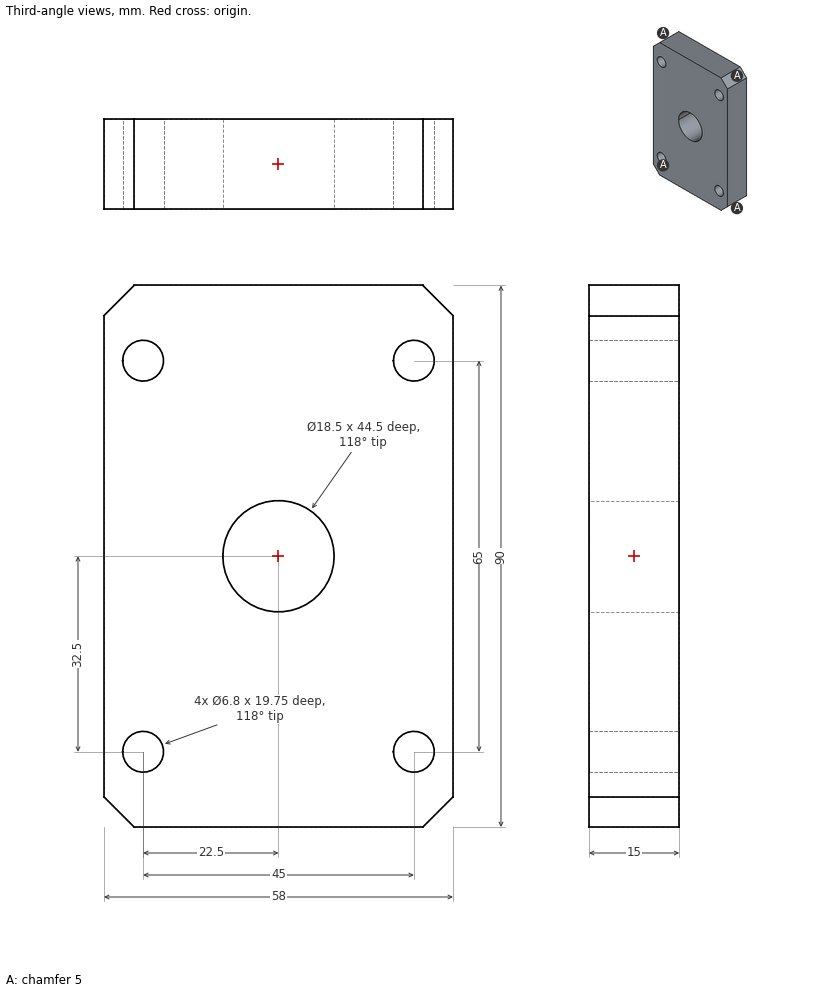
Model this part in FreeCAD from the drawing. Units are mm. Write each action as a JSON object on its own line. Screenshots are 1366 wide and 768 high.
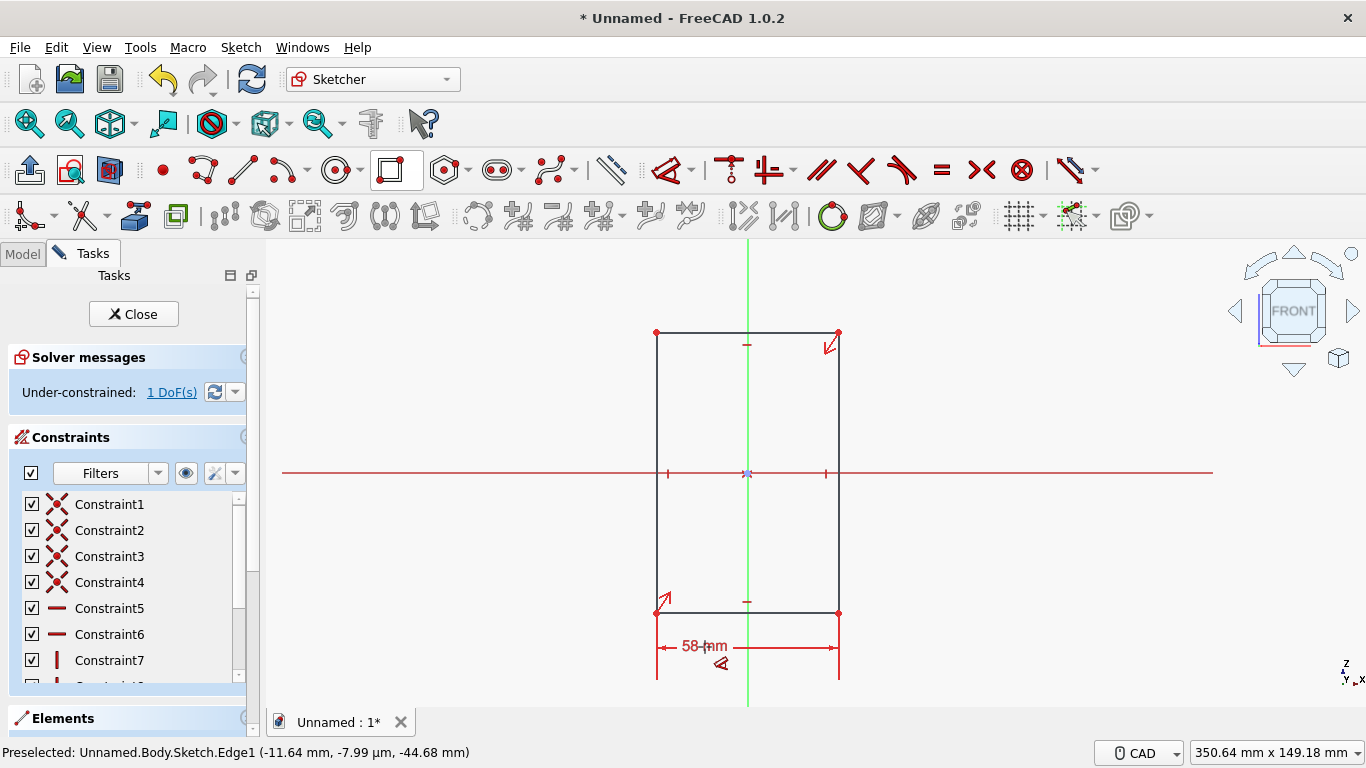
{"action": "left_click", "coordinate": [839, 529]}
{"action": "left_click", "coordinate": [873, 409]}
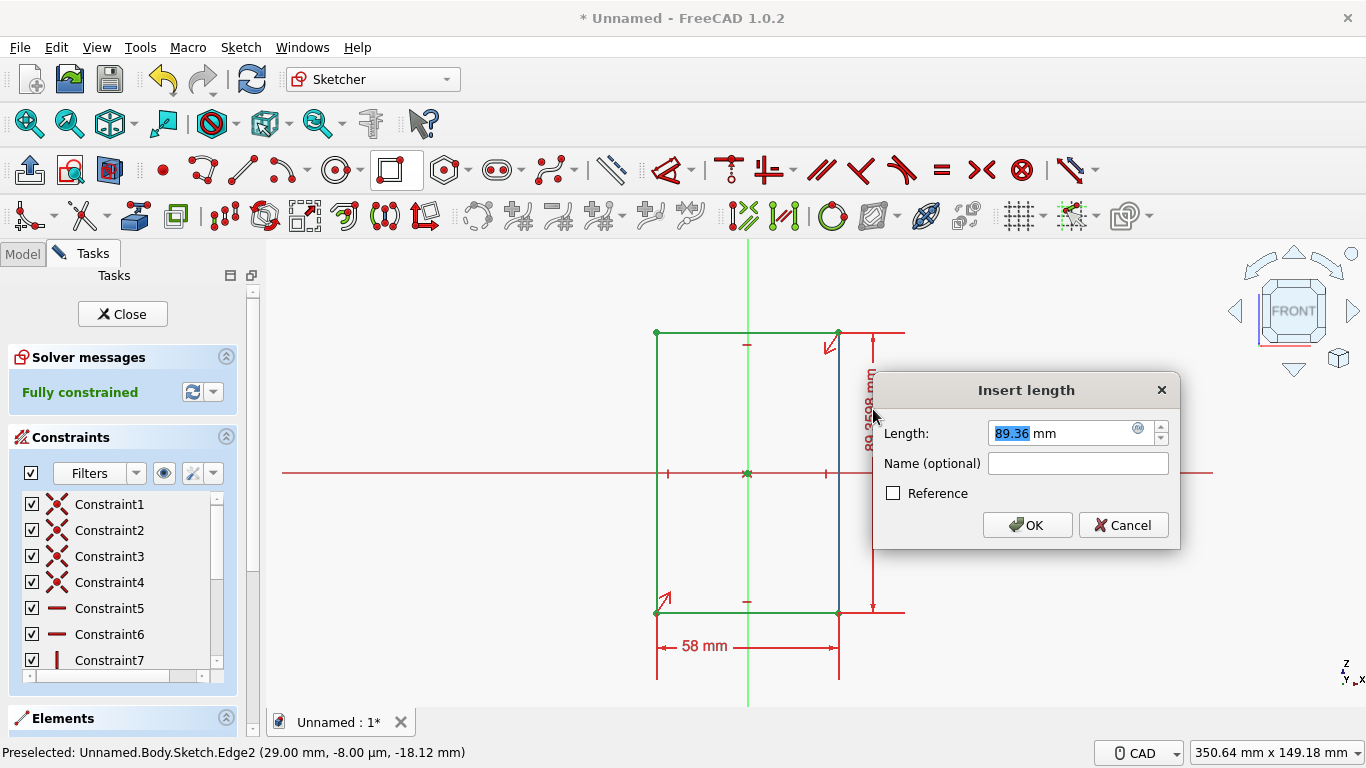
{"action": "type", "text": "90"}
{"action": "key", "text": "Return"}
{"action": "key", "text": "Escape"}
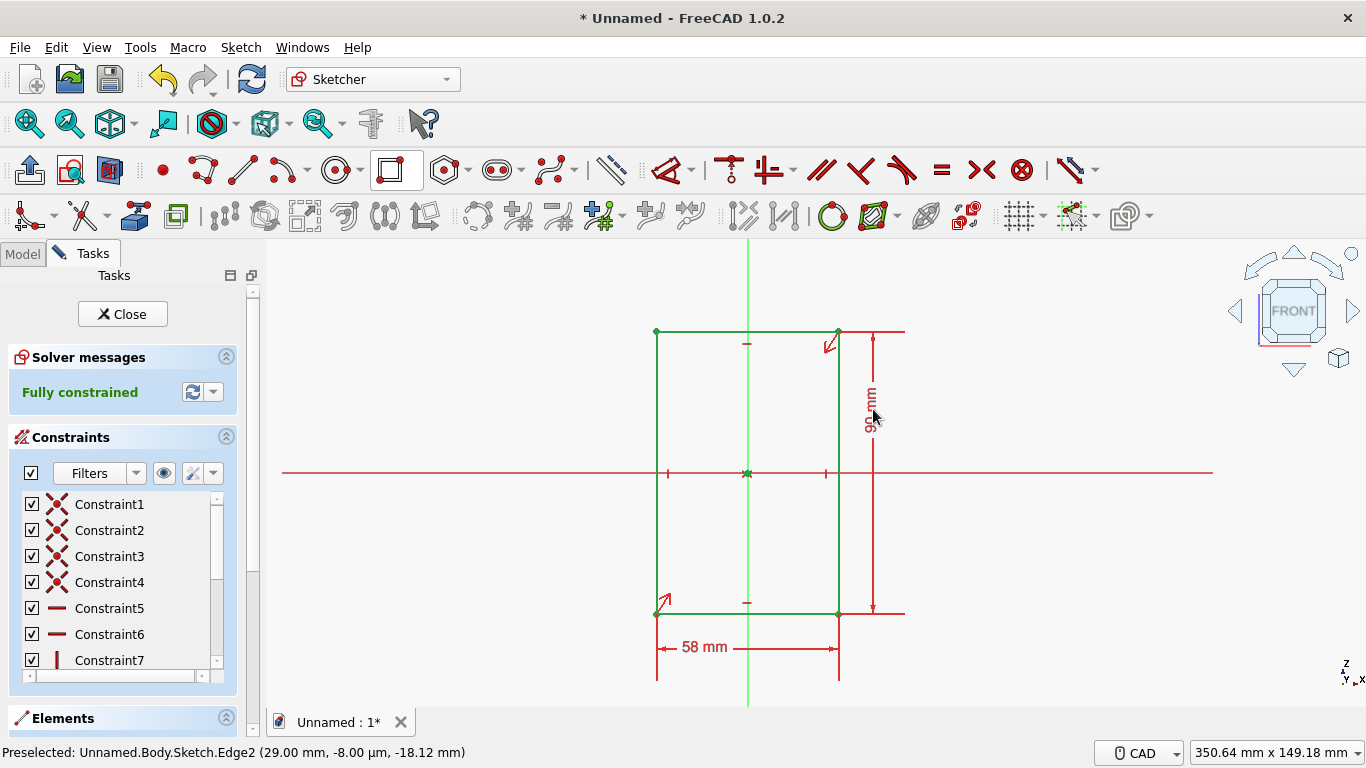
{"action": "left_click", "coordinate": [123, 314]}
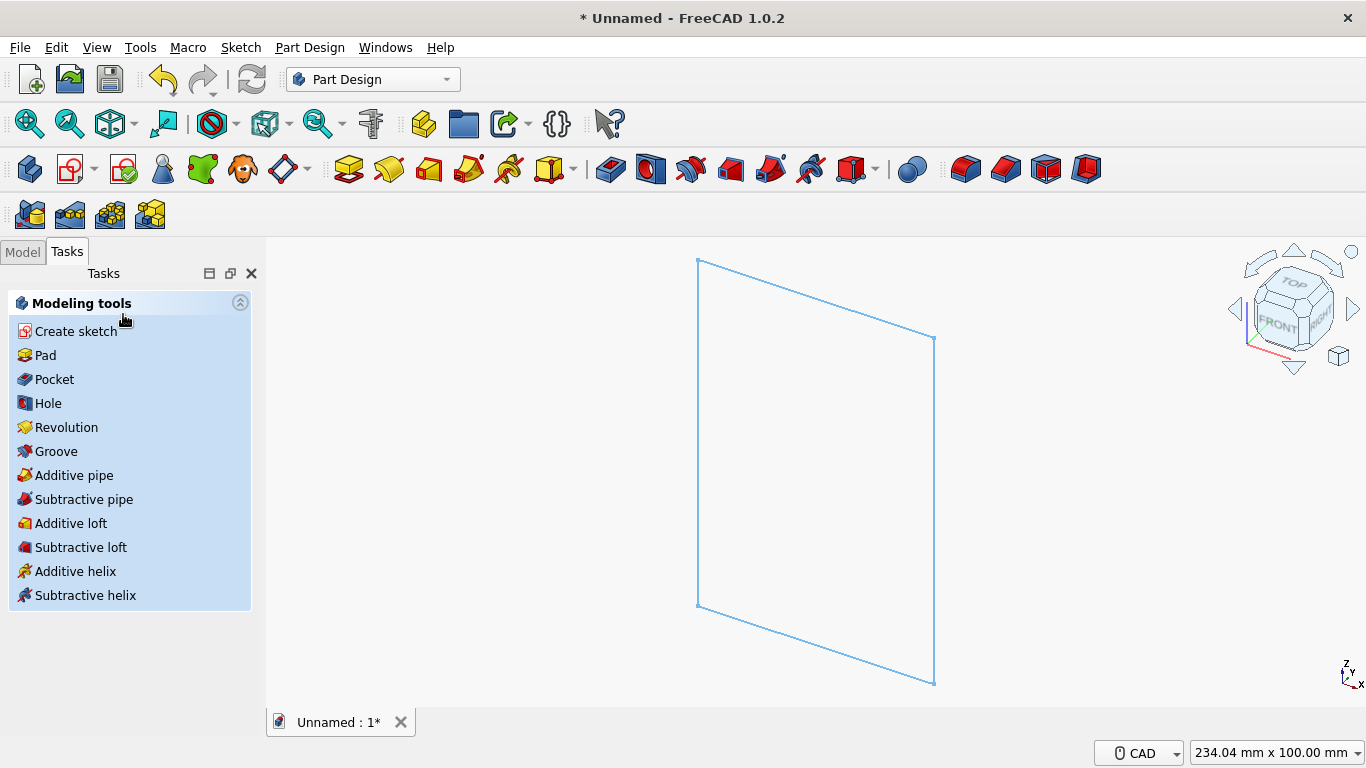
{"action": "left_click", "coordinate": [350, 170]}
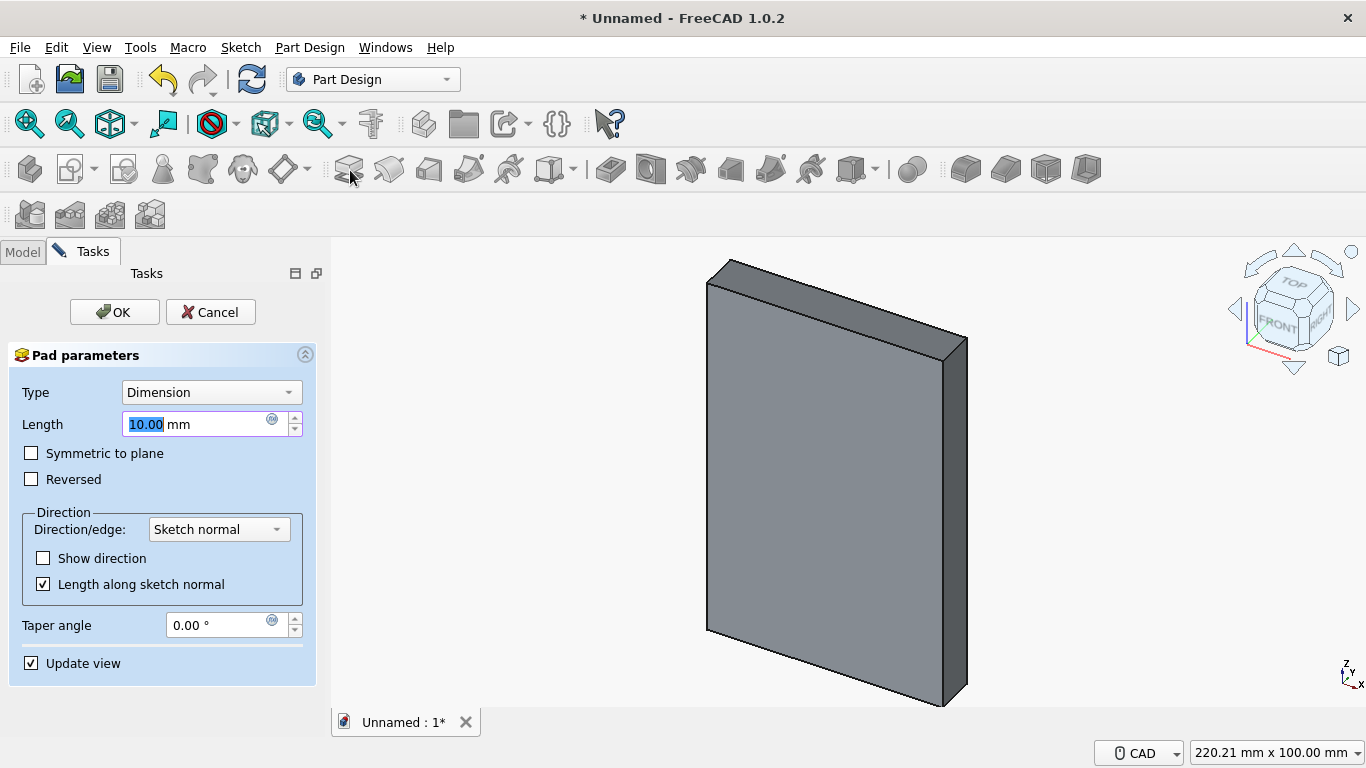
{"action": "type", "text": "15"}
{"action": "key", "text": "Tab"}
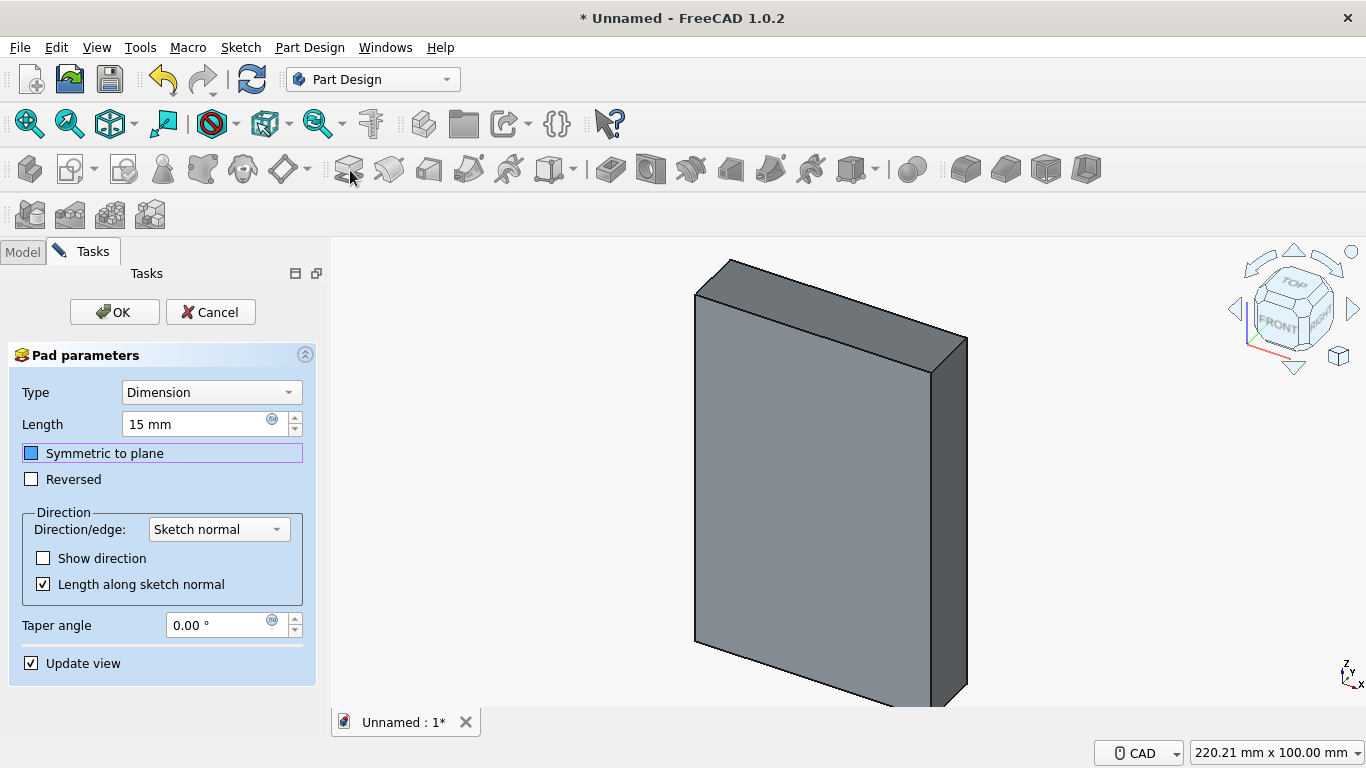
{"action": "left_click", "coordinate": [30, 453]}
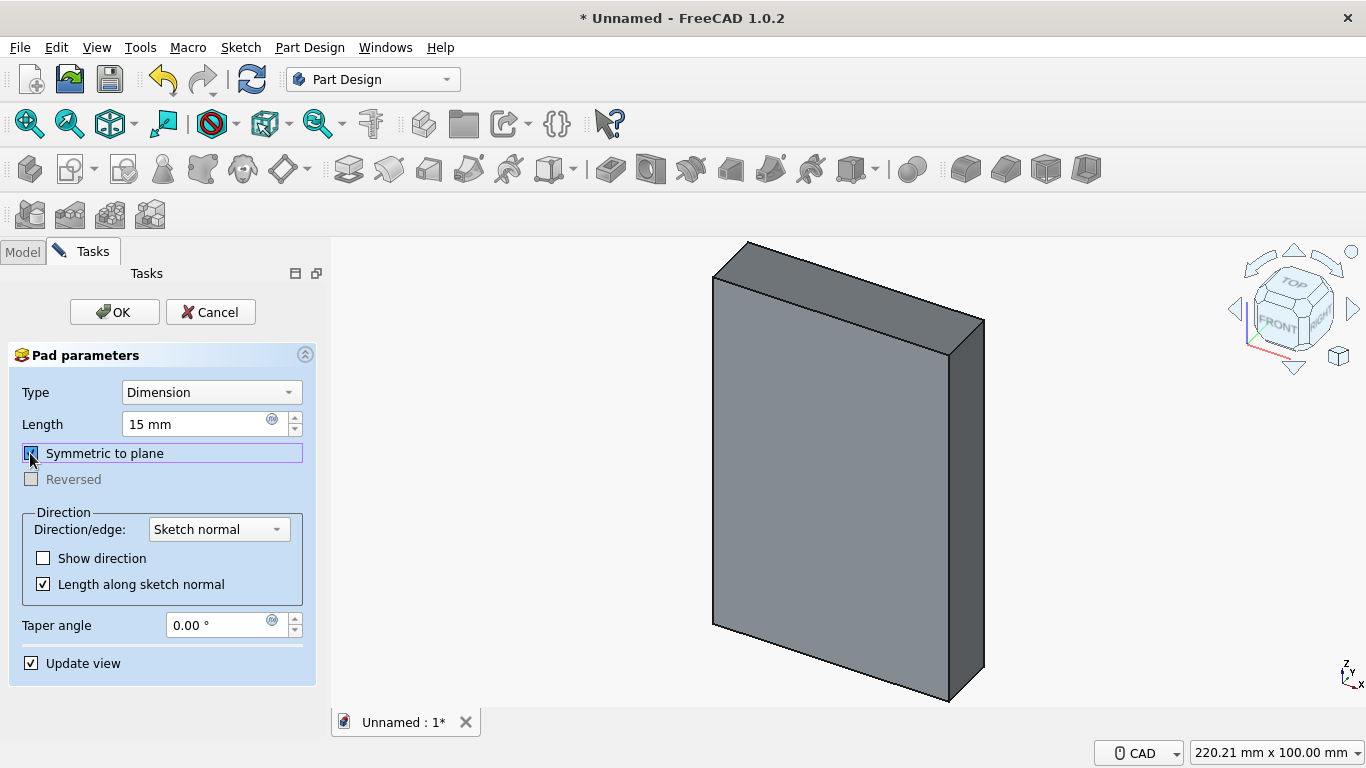
{"action": "left_click", "coordinate": [115, 312]}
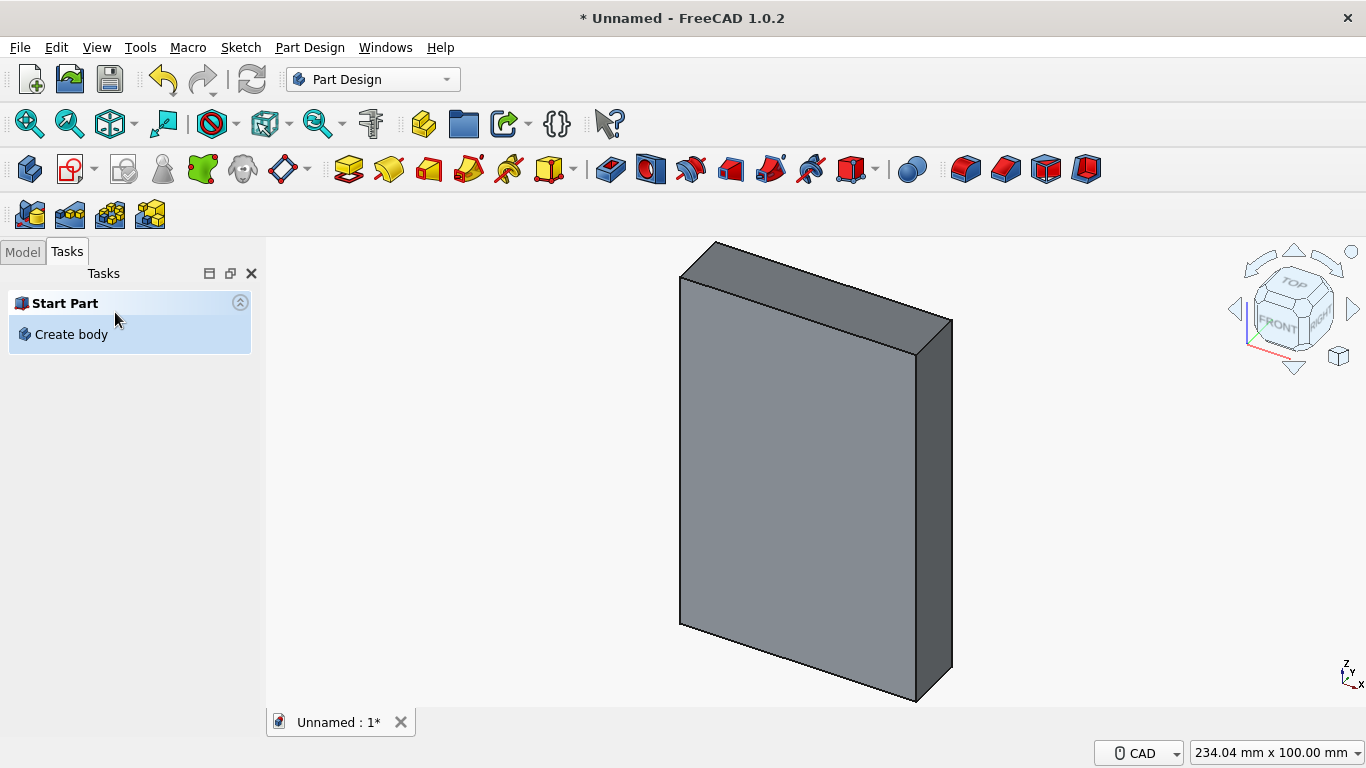
{"action": "left_click", "coordinate": [798, 439]}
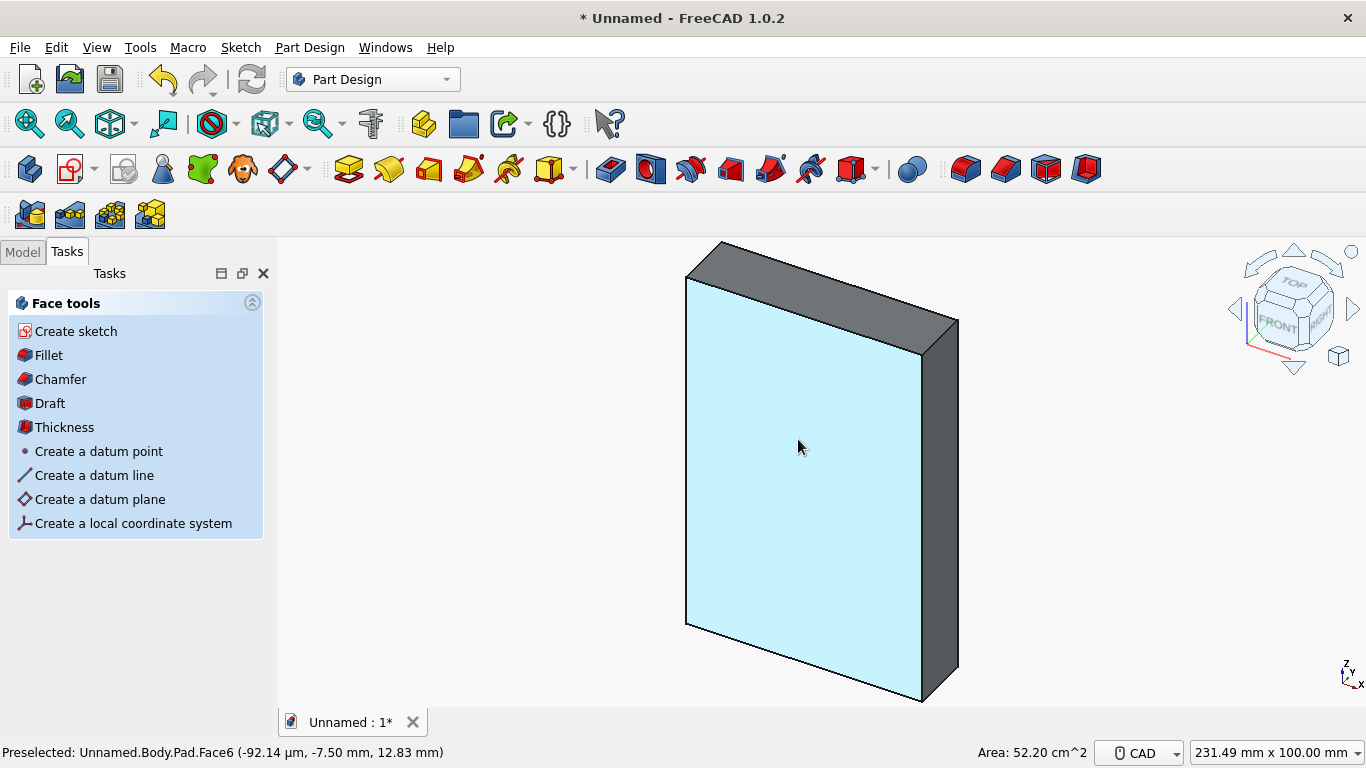
{"action": "left_click", "coordinate": [70, 170]}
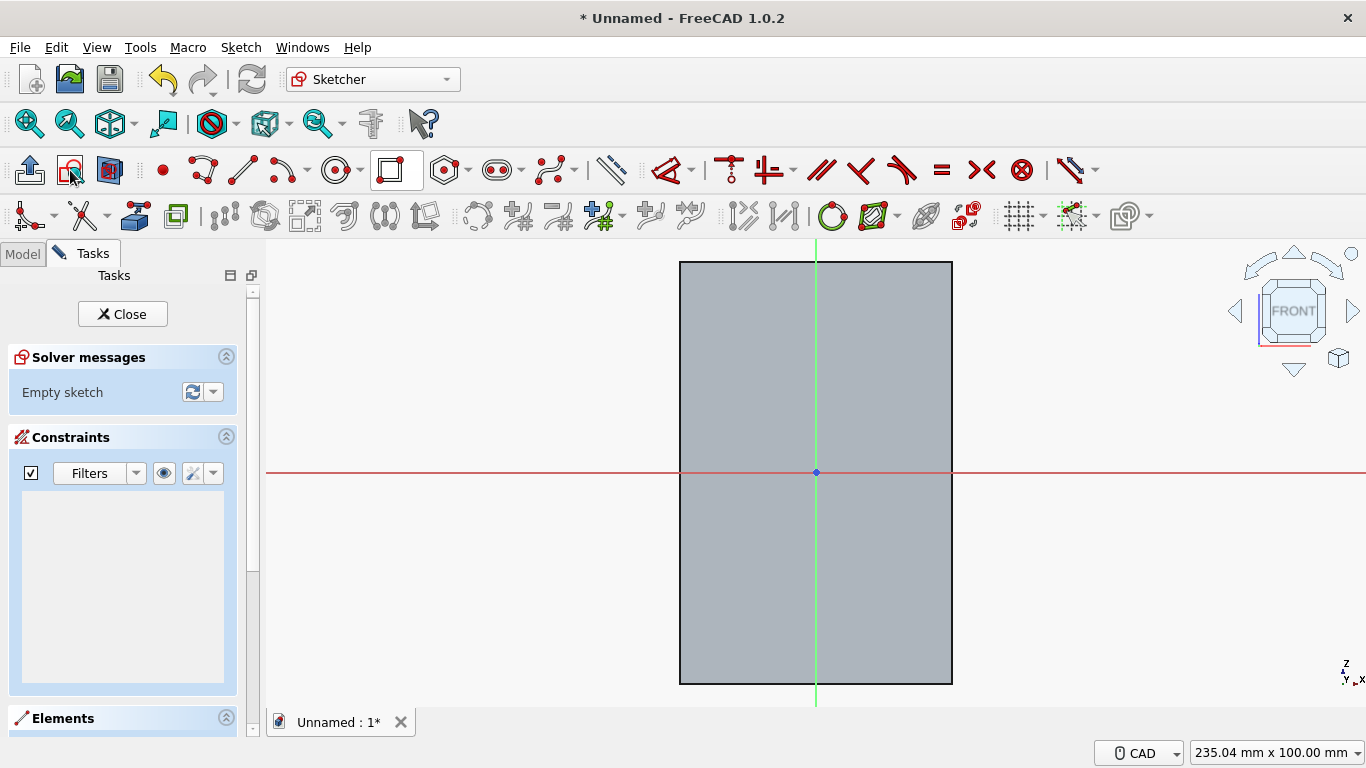
{"action": "key", "text": "g c"}